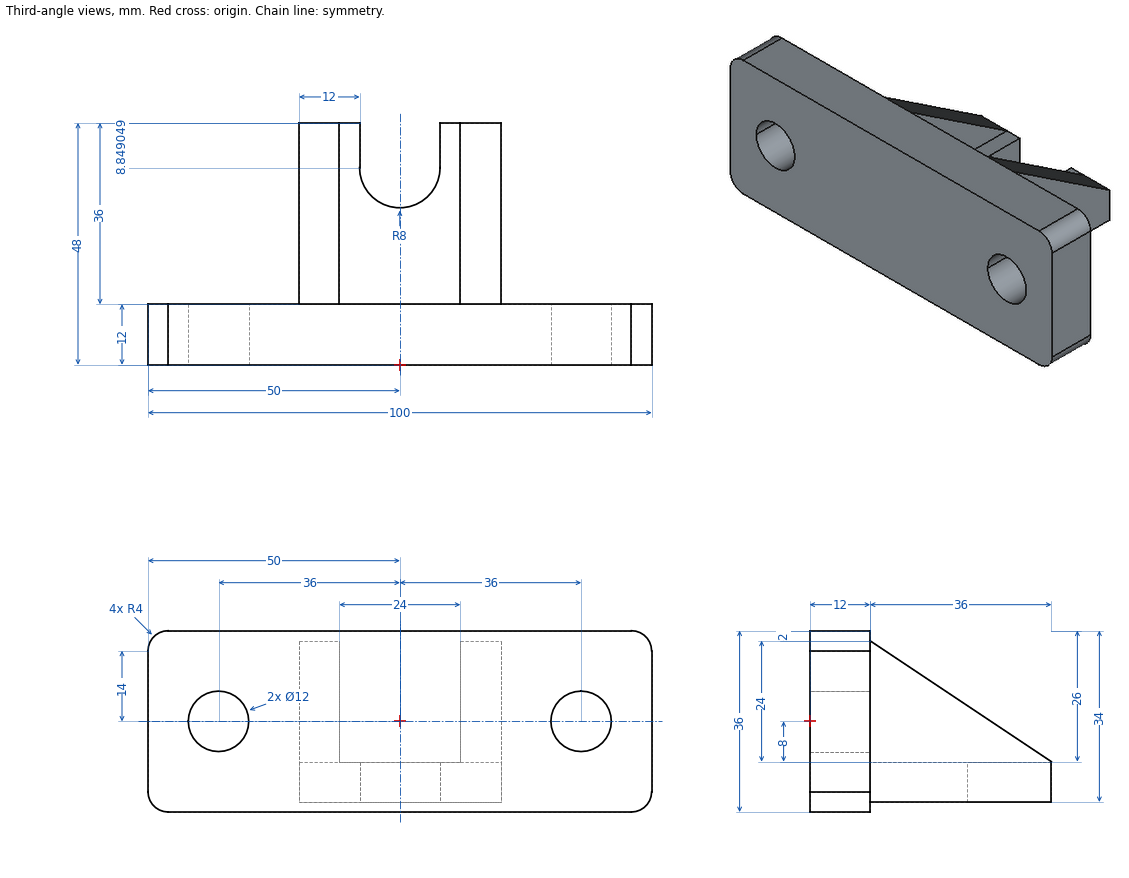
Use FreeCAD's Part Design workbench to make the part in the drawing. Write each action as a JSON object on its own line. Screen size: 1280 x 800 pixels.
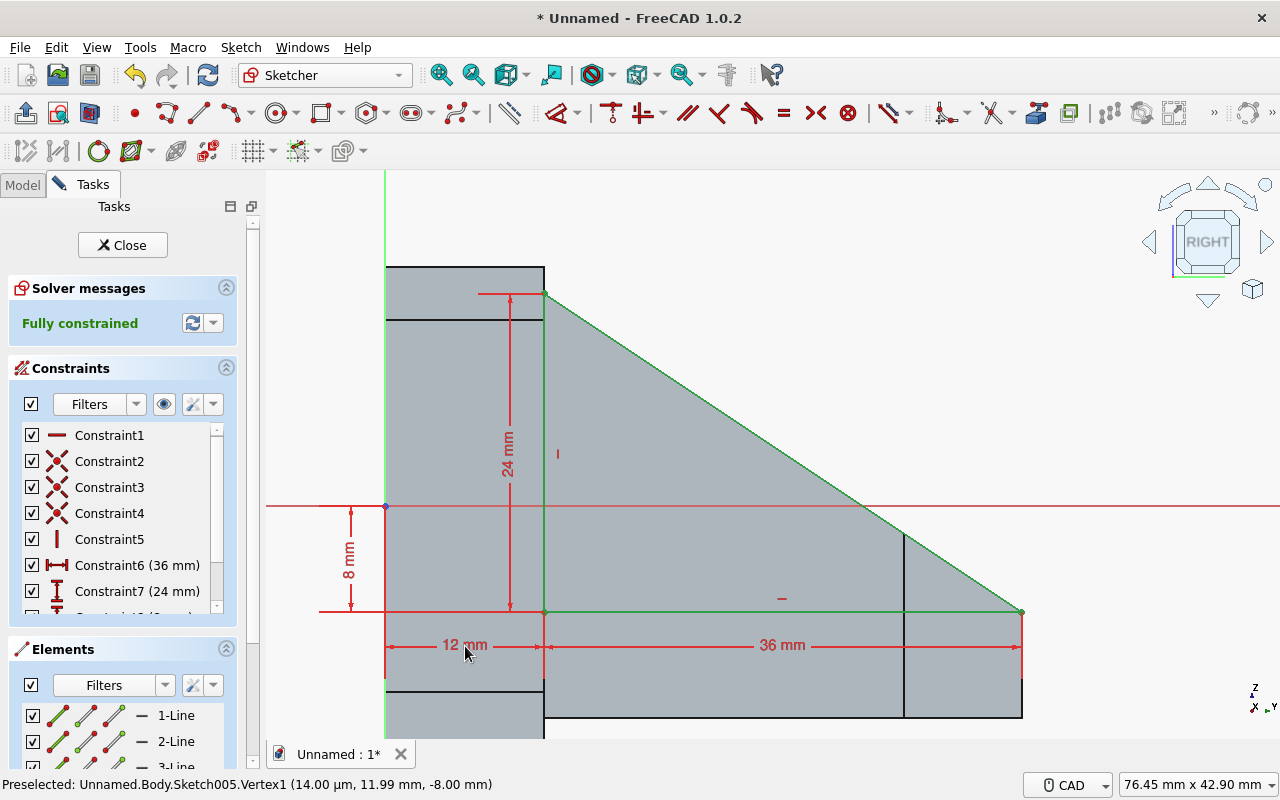
{"action": "left_click", "coordinate": [123, 245]}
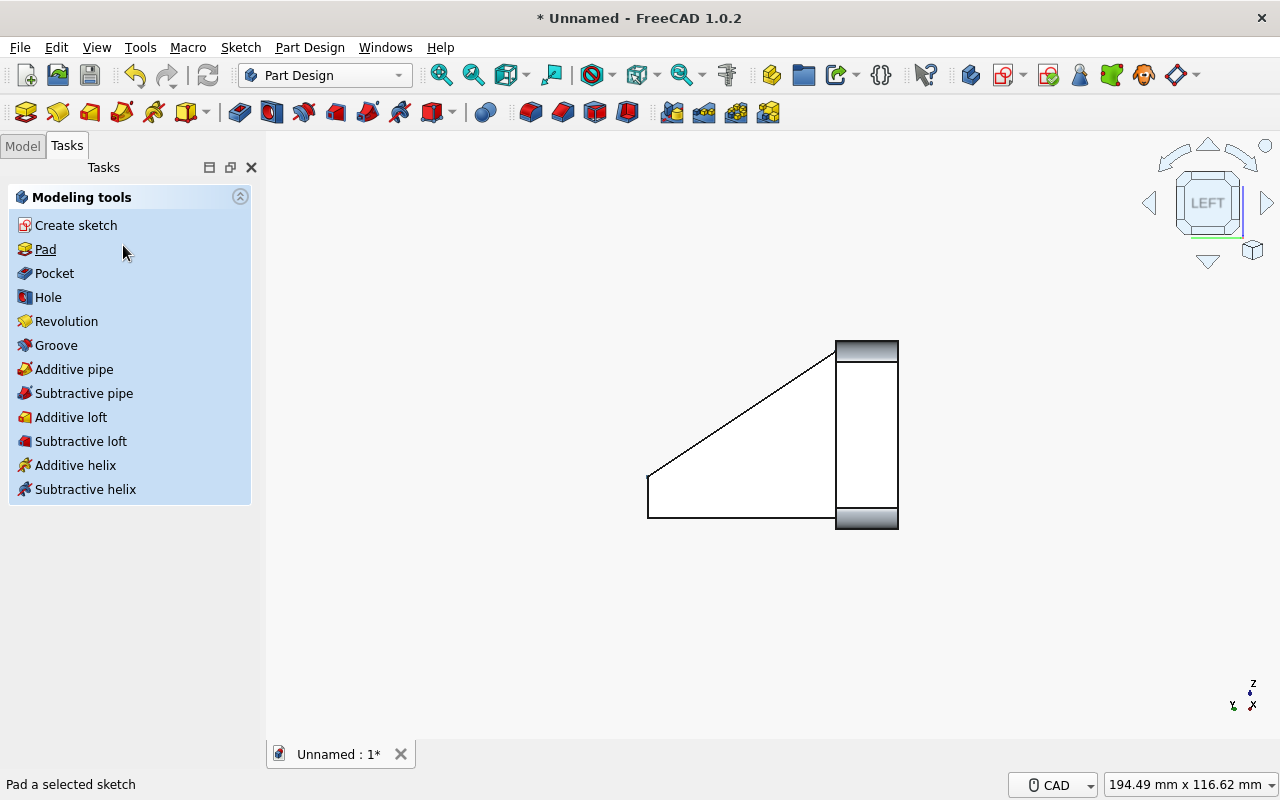
{"action": "left_click", "coordinate": [240, 112]}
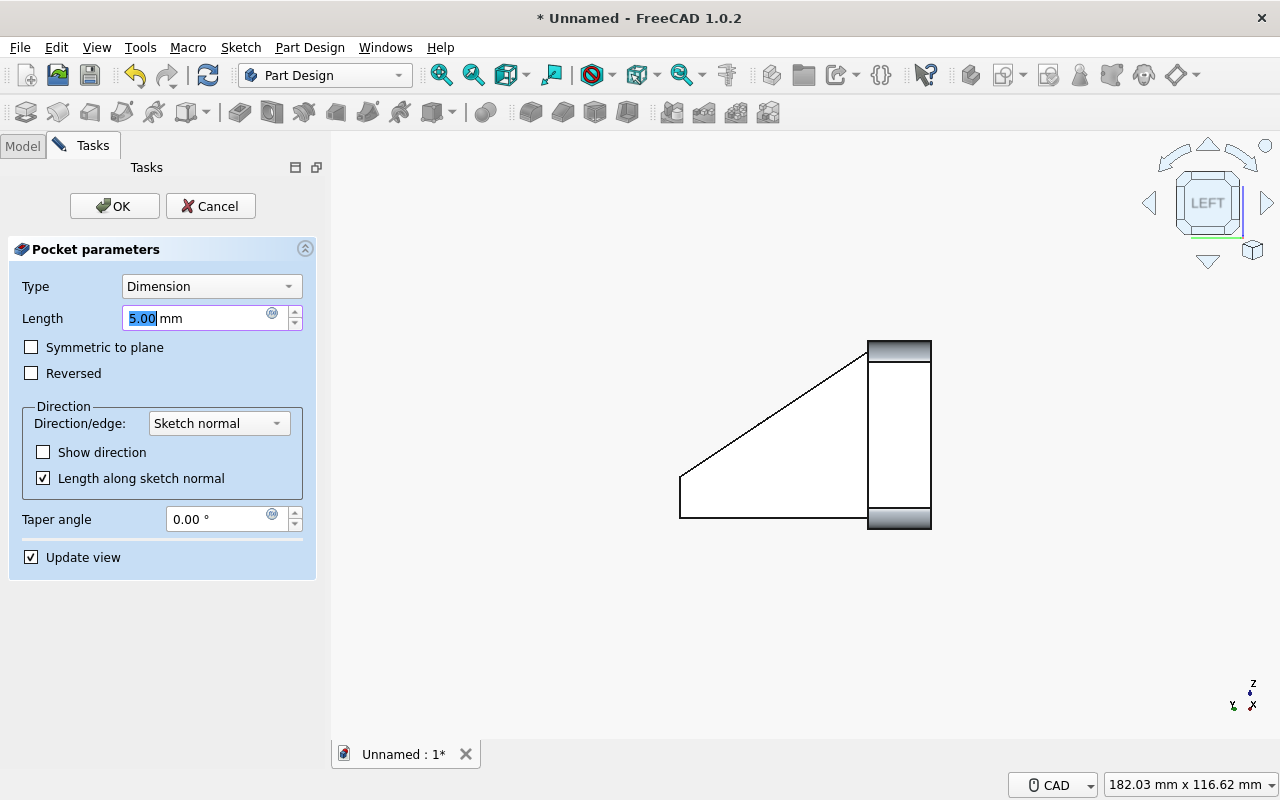
{"action": "type", "text": "24"}
{"action": "key", "text": "Tab"}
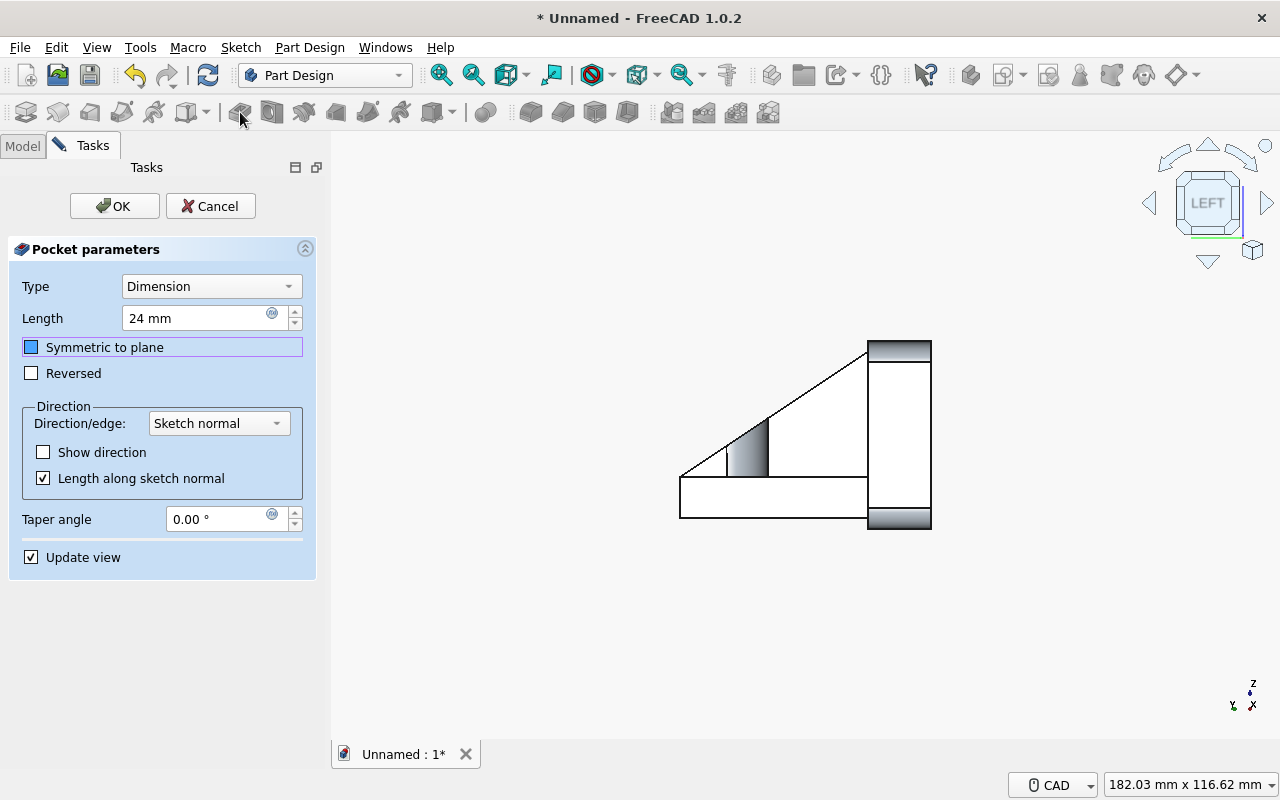
{"action": "left_click", "coordinate": [30, 347]}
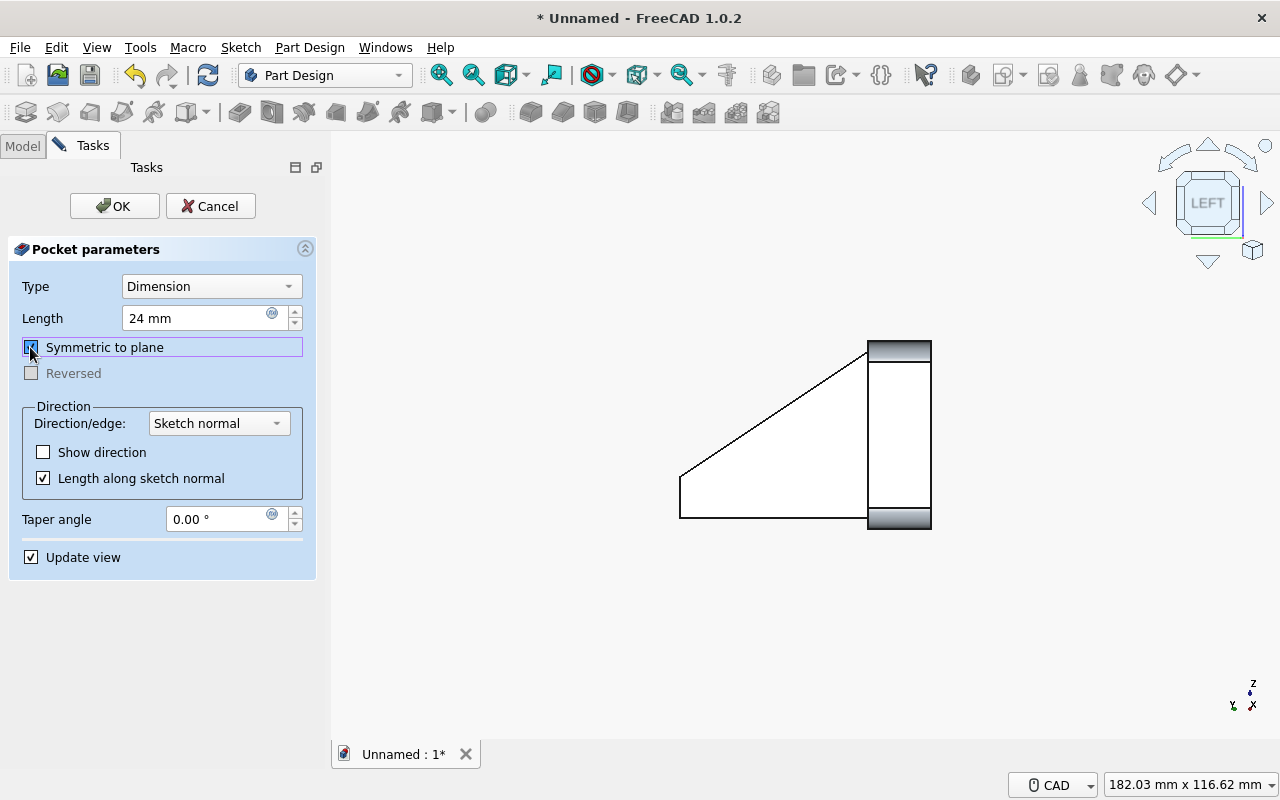
{"action": "left_click", "coordinate": [115, 206]}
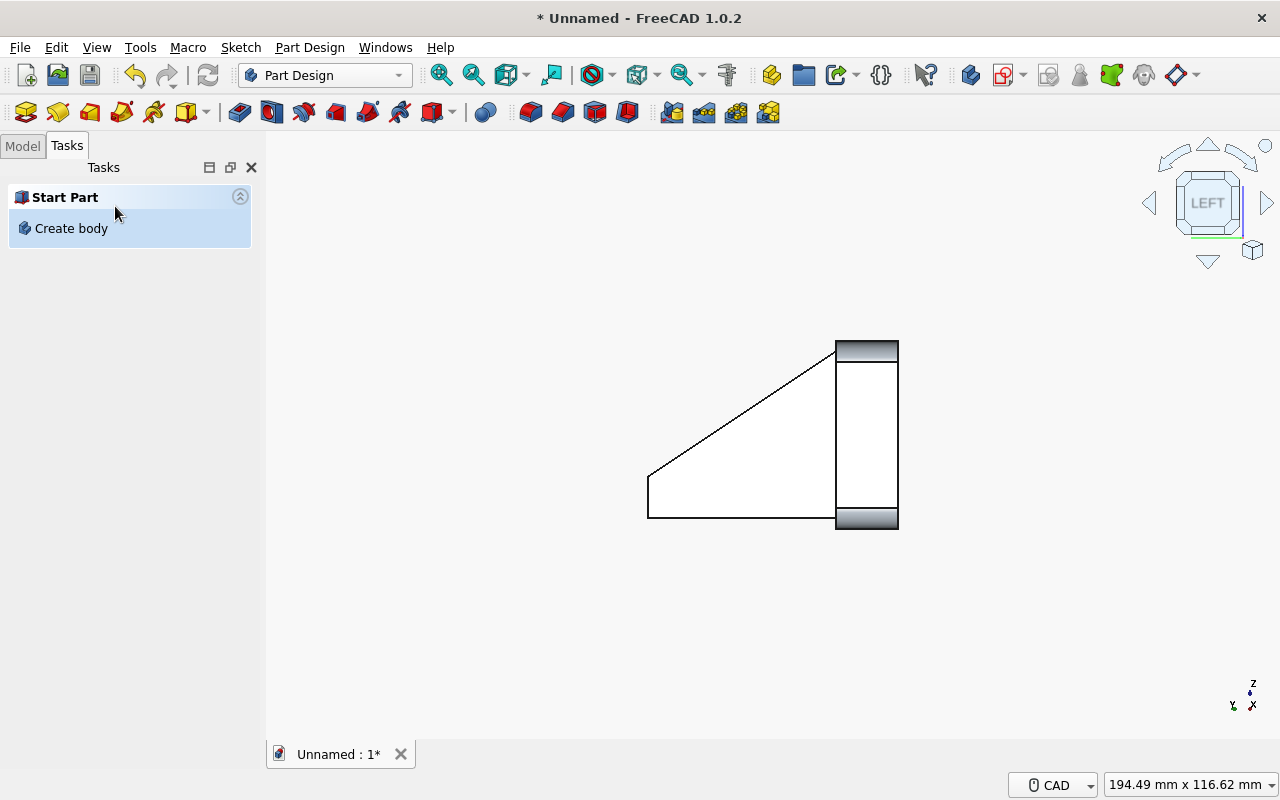
{"action": "key", "text": "0"}